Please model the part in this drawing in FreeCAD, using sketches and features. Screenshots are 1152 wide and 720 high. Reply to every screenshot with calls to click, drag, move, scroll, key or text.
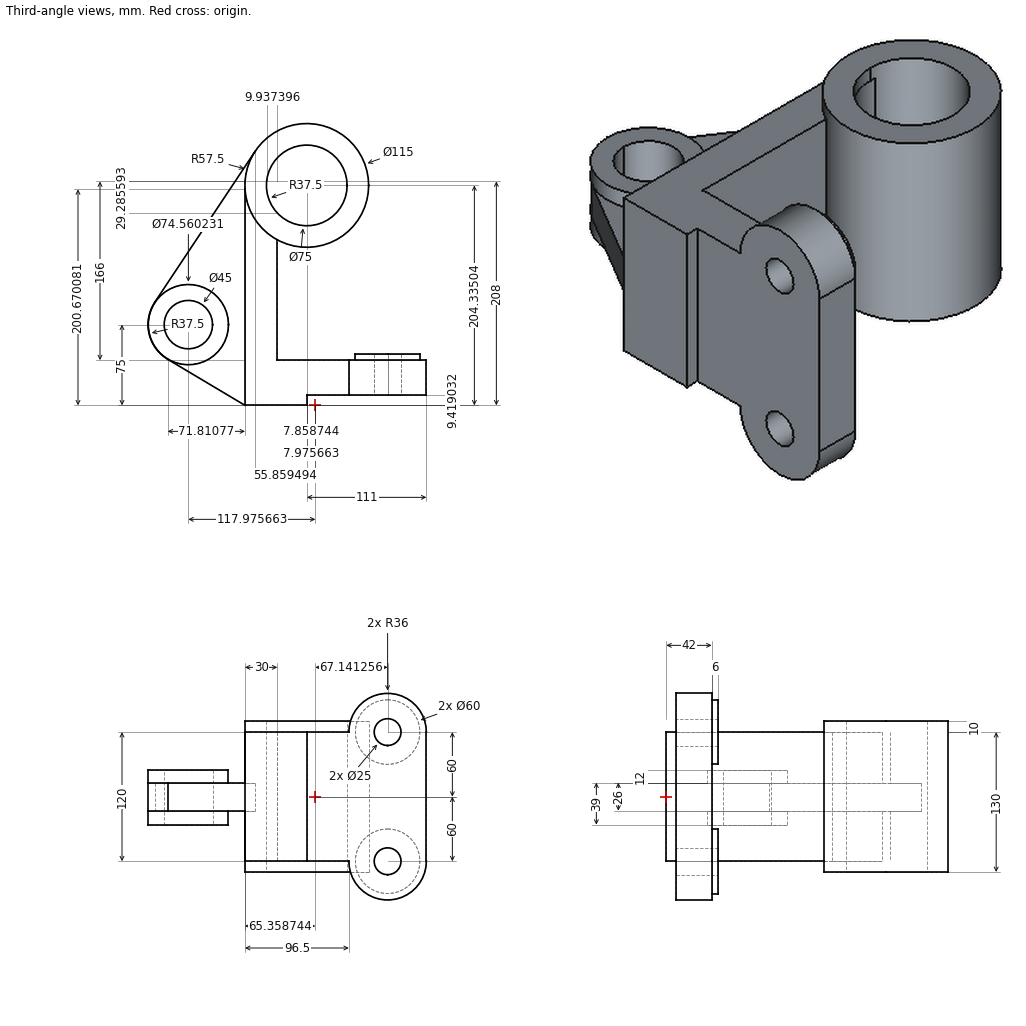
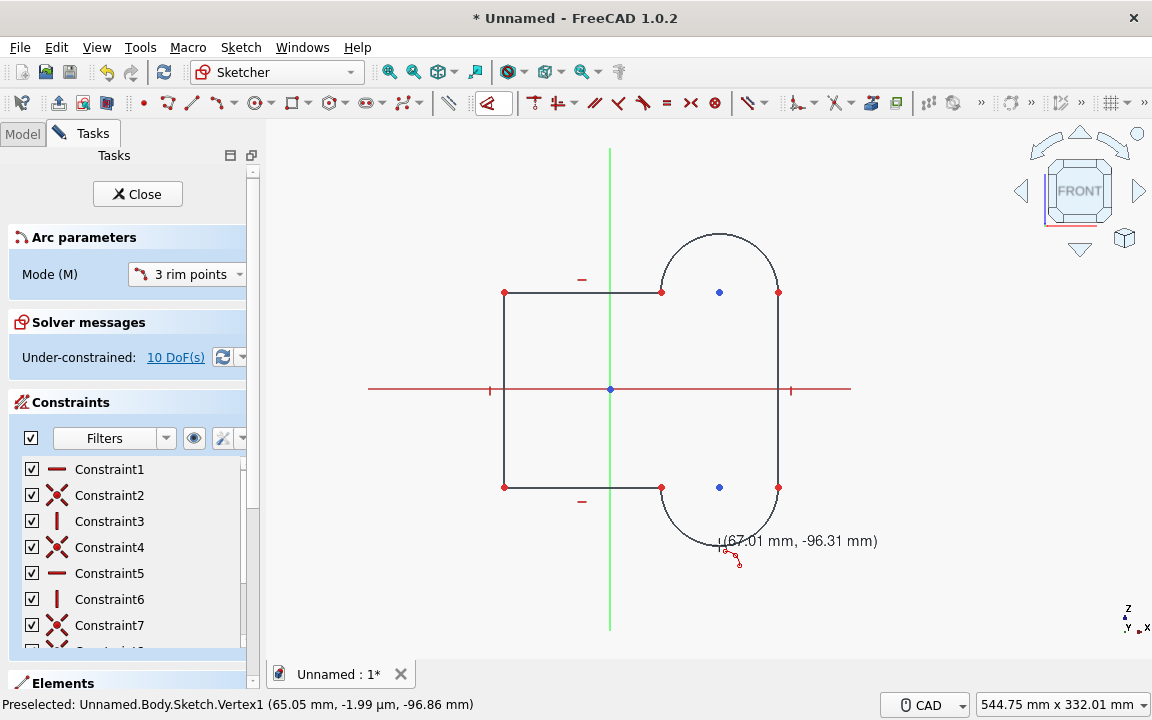
click(256, 104)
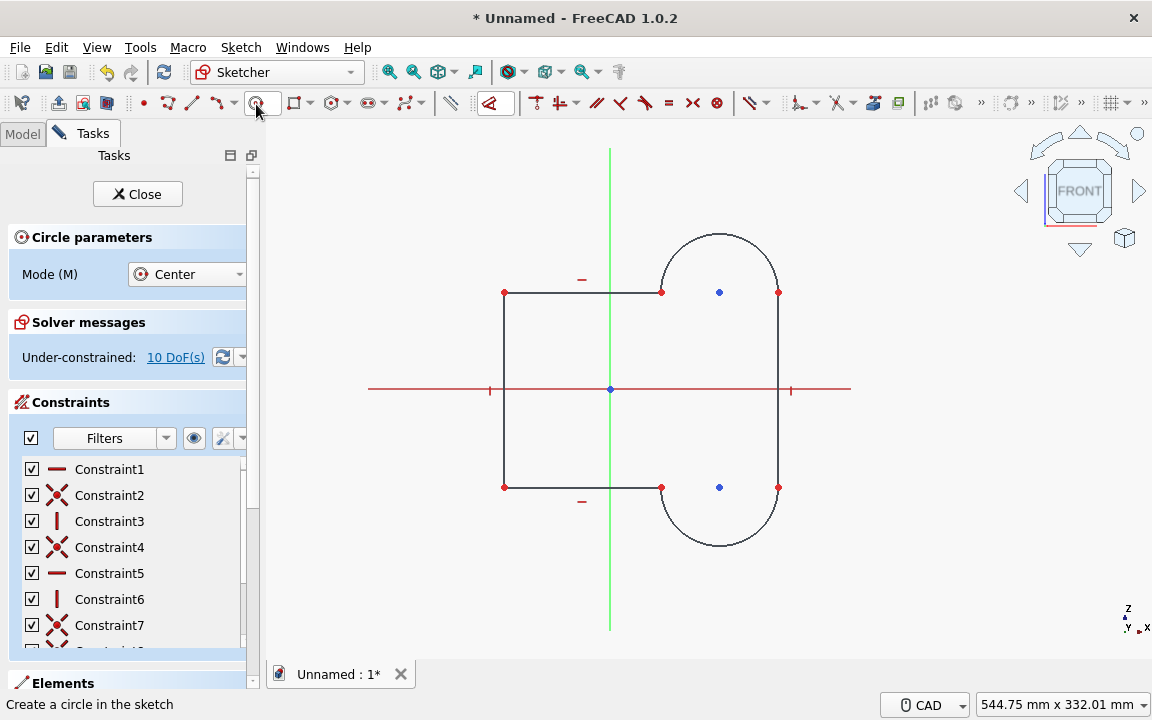
click(719, 292)
move(734, 277)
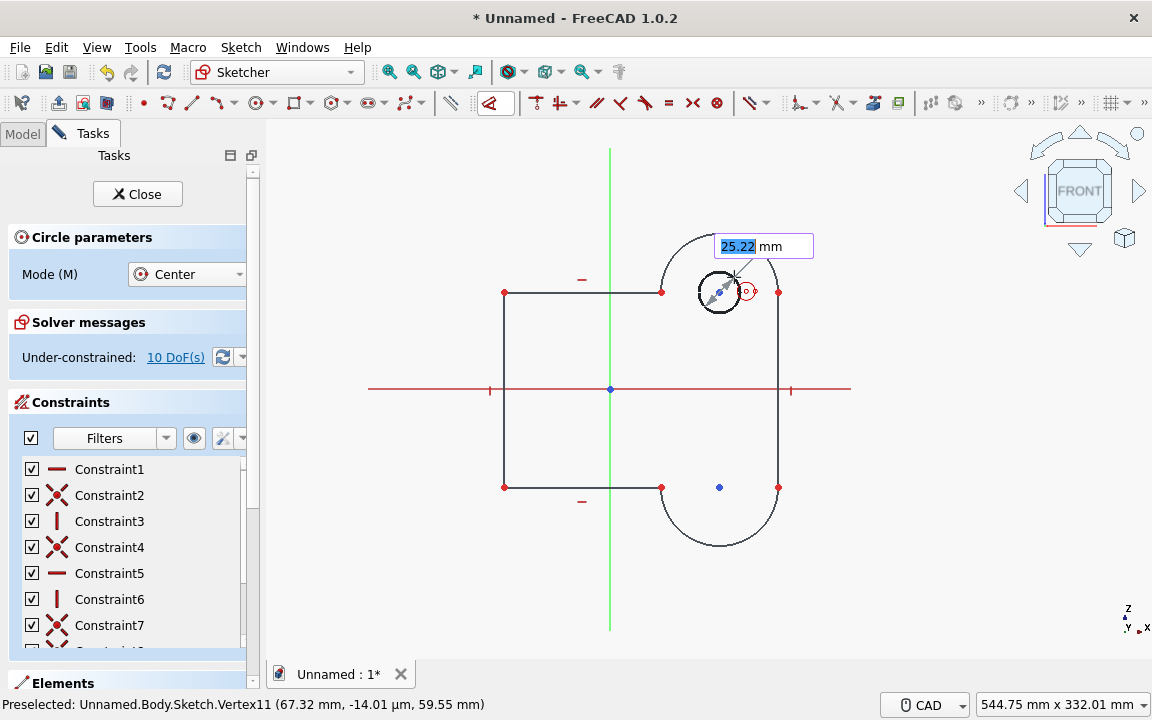
text(25)
key(Return)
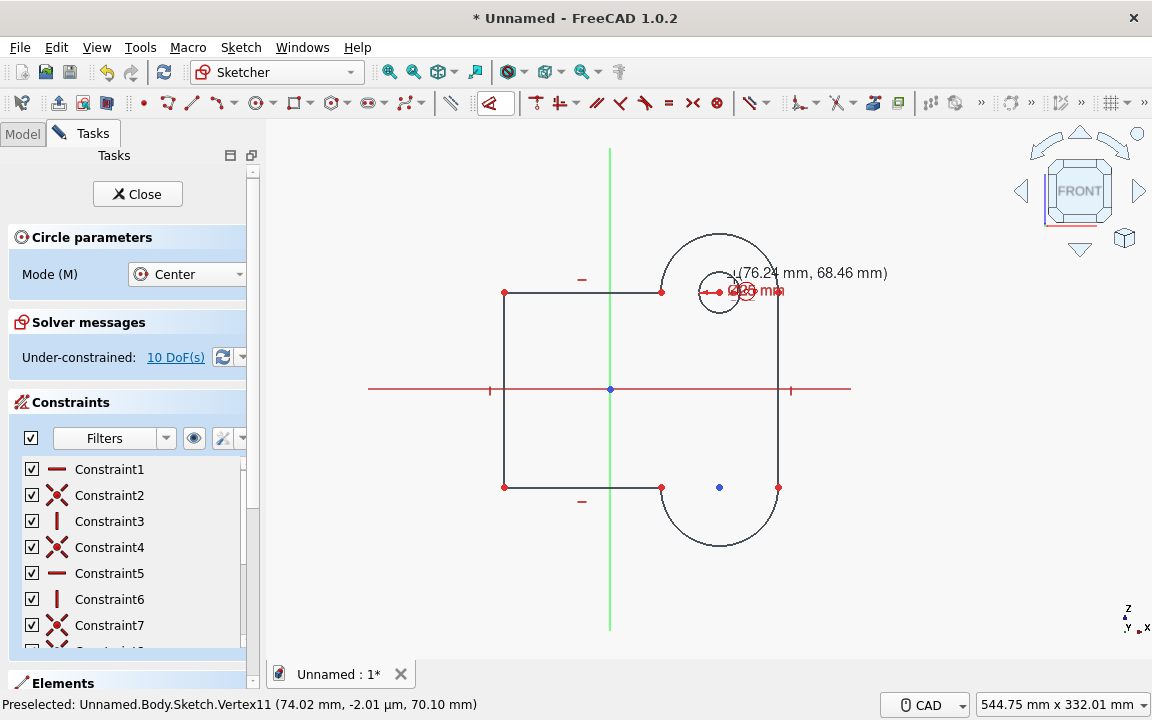
click(719, 487)
move(734, 473)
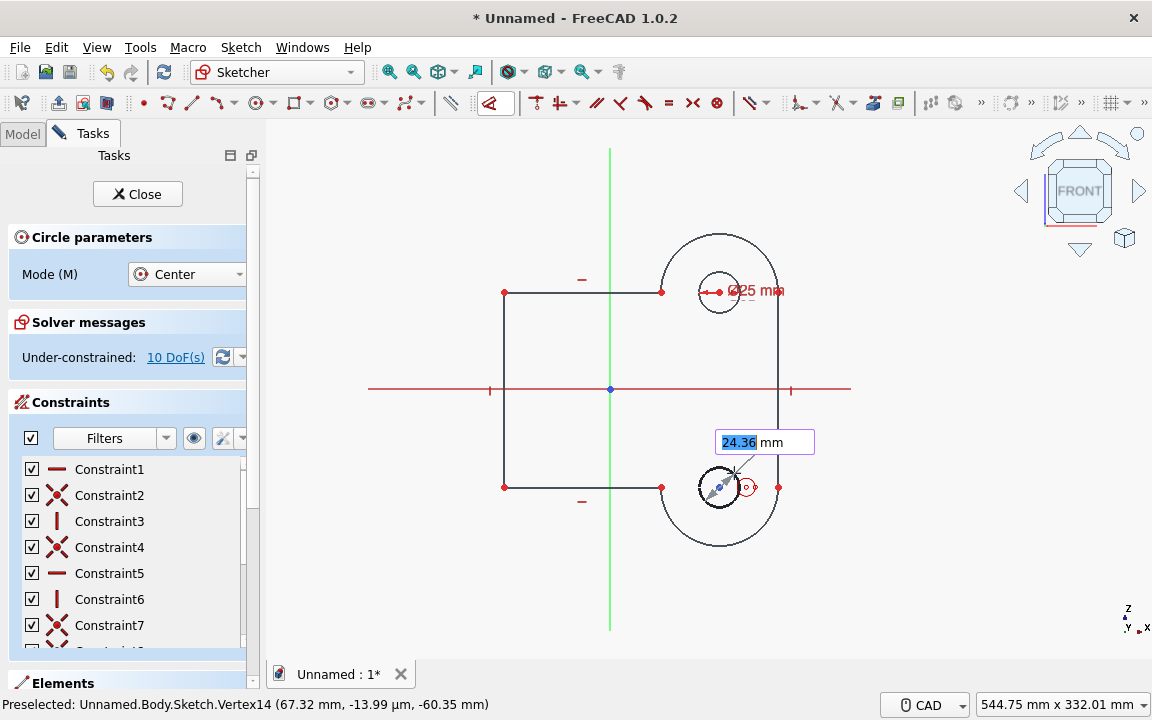
text(25)
key(Return)
key(Escape)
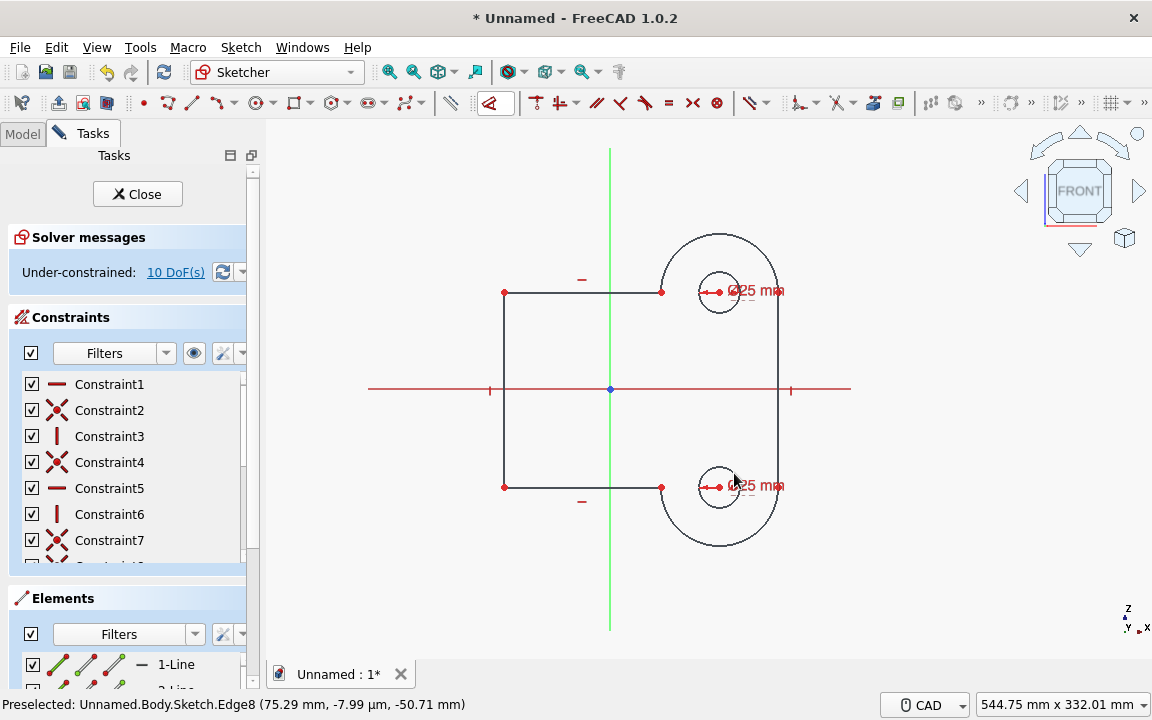
click(778, 351)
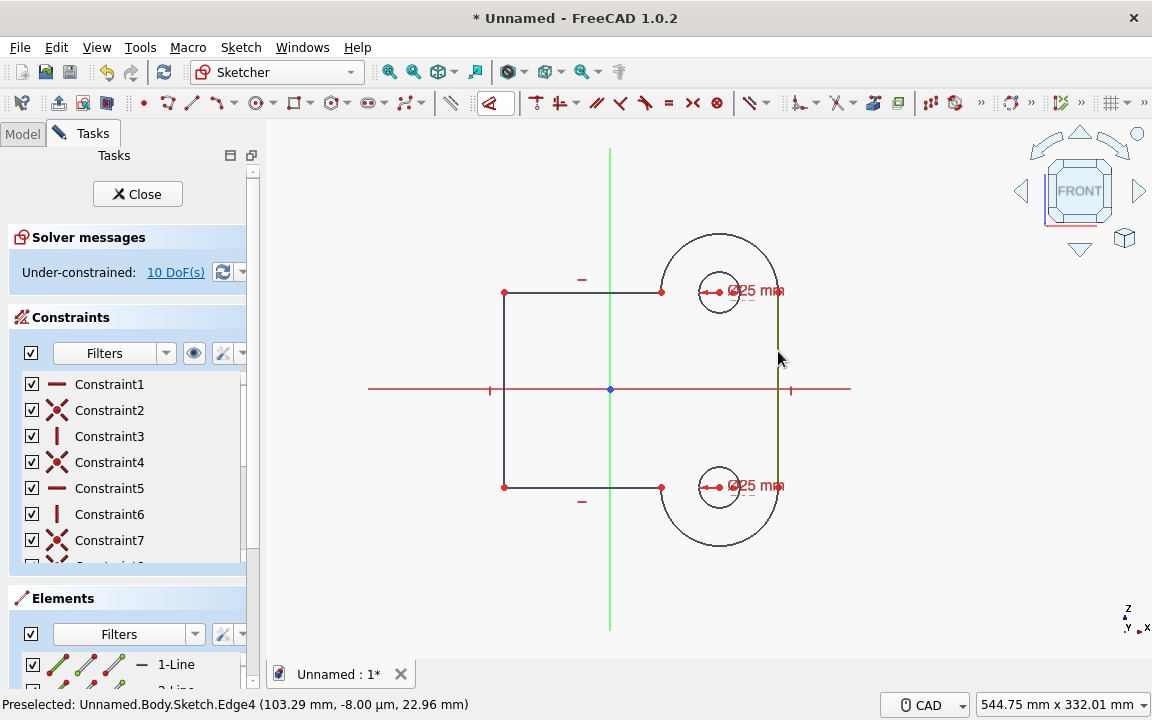
click(754, 245)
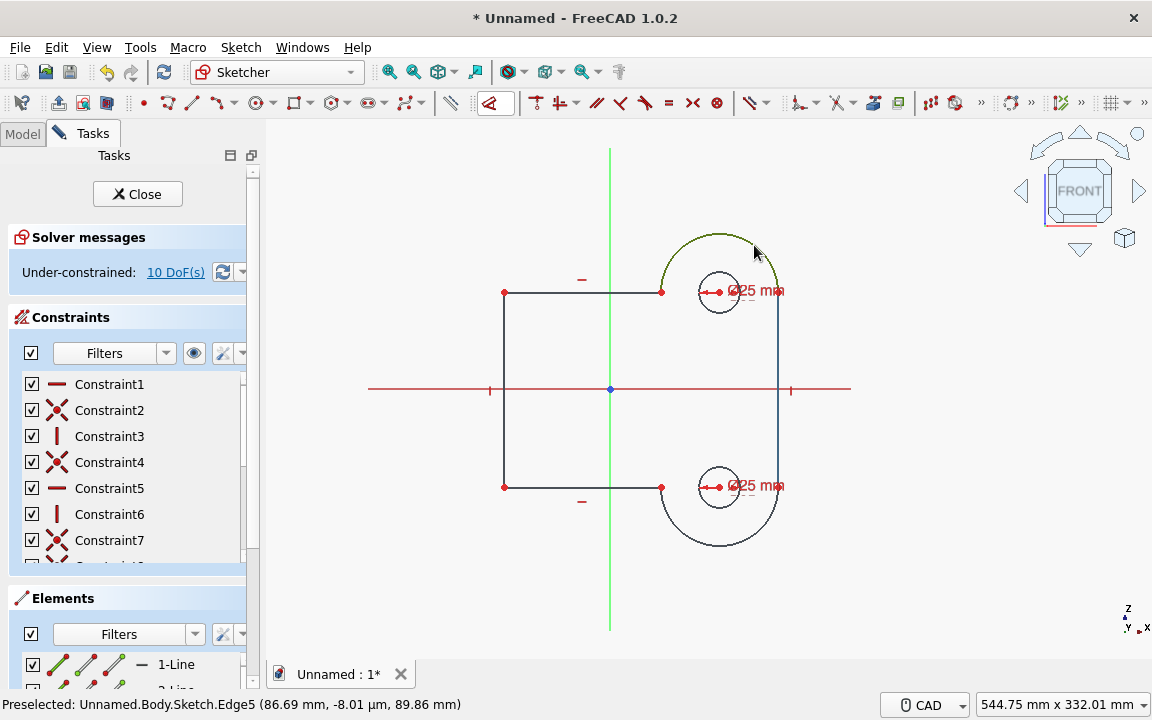
click(646, 104)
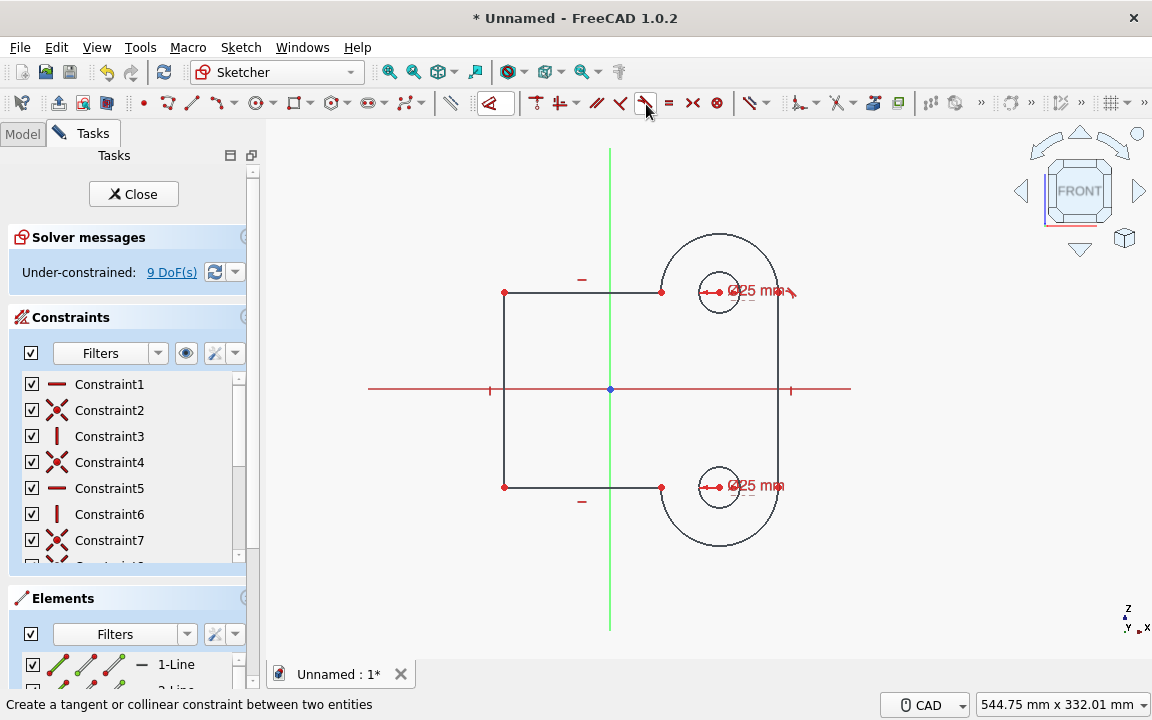
click(778, 351)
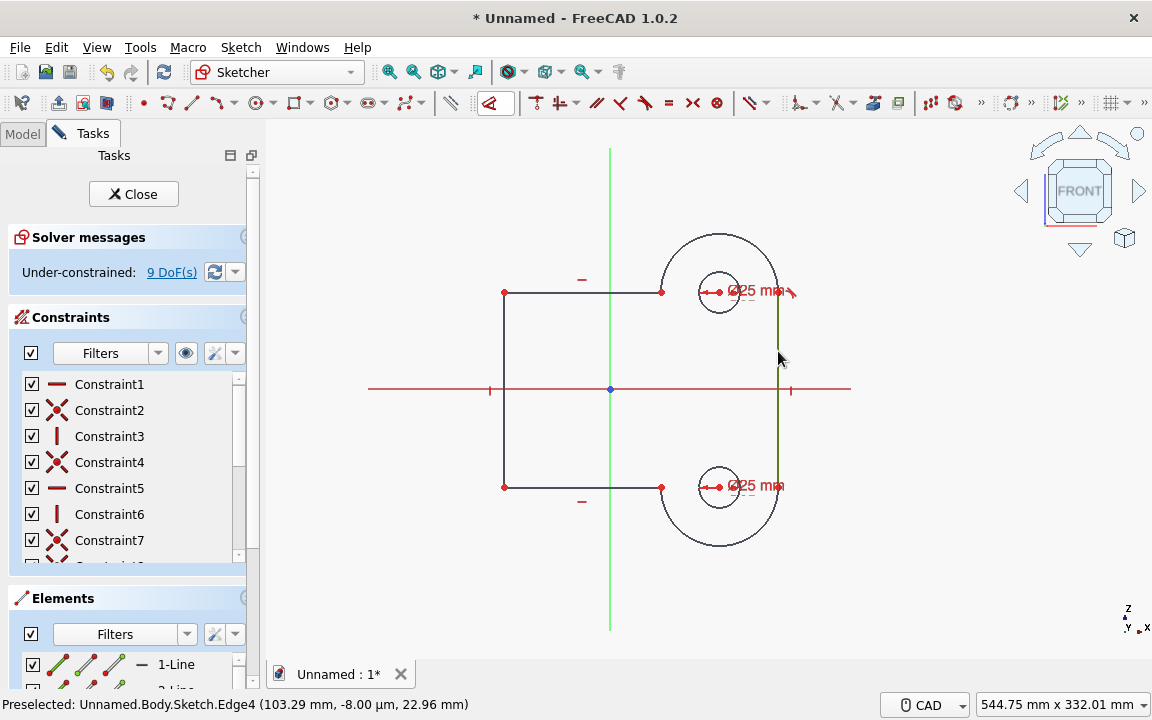
click(685, 535)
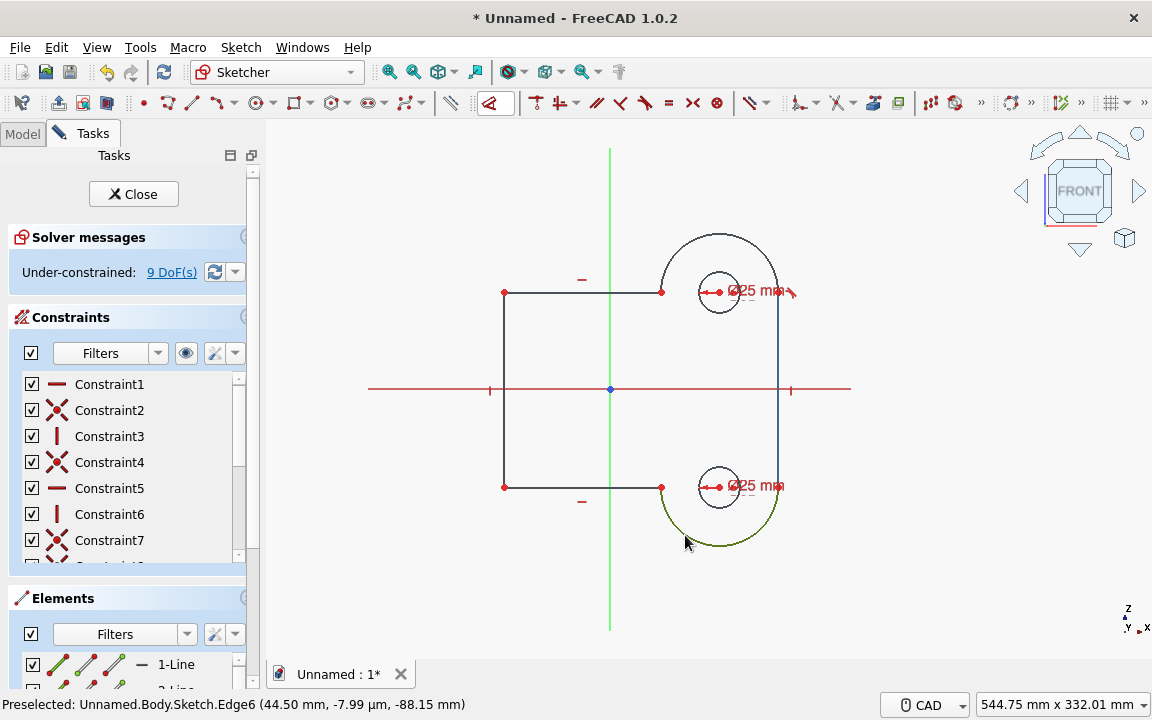
click(646, 104)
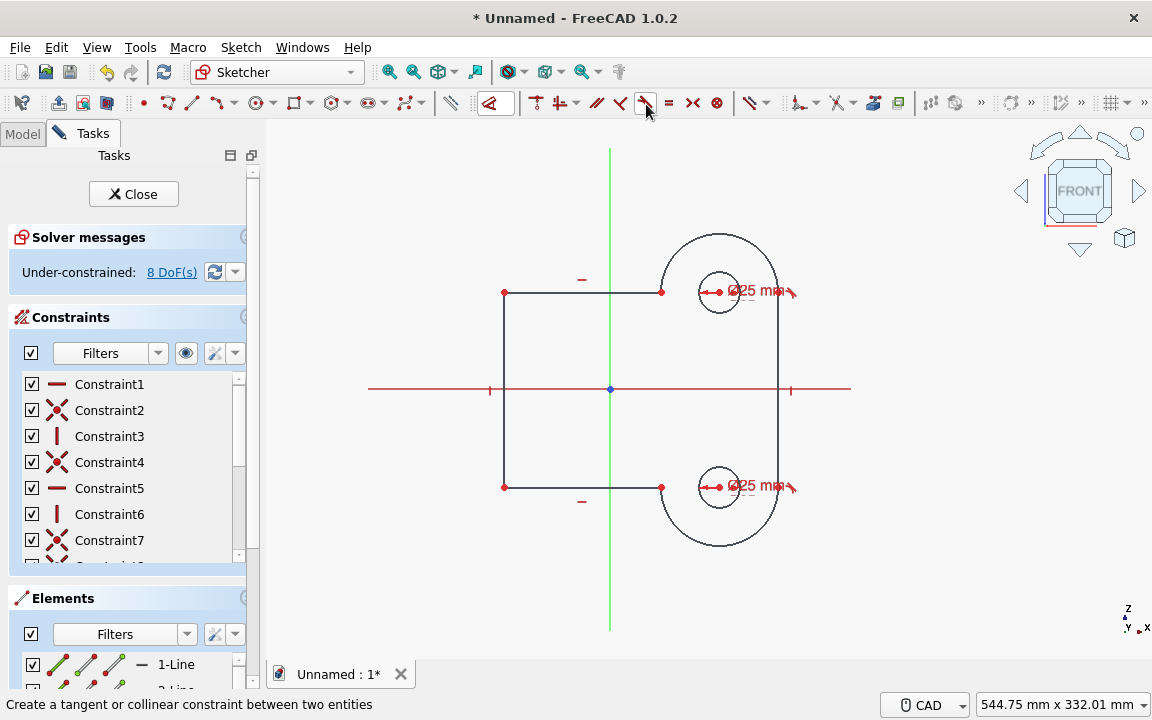
click(754, 245)